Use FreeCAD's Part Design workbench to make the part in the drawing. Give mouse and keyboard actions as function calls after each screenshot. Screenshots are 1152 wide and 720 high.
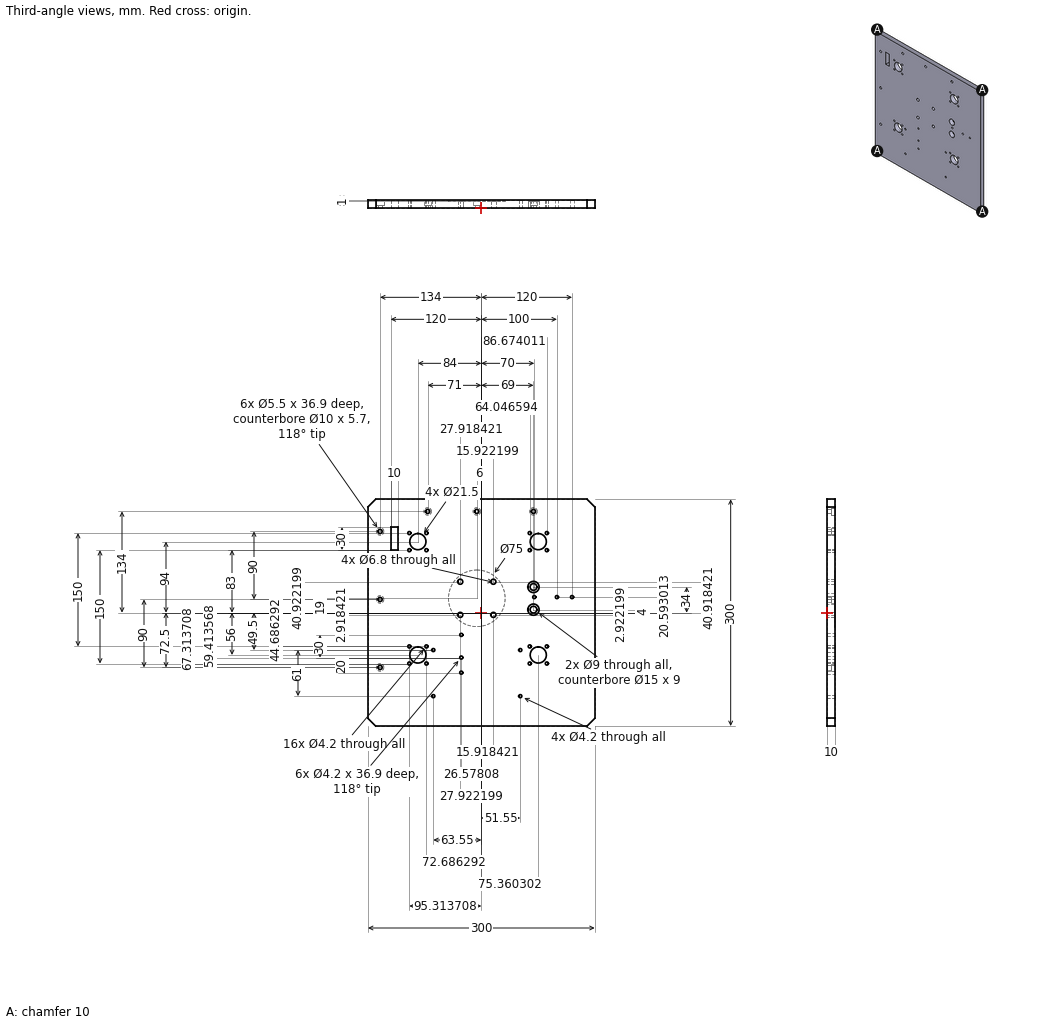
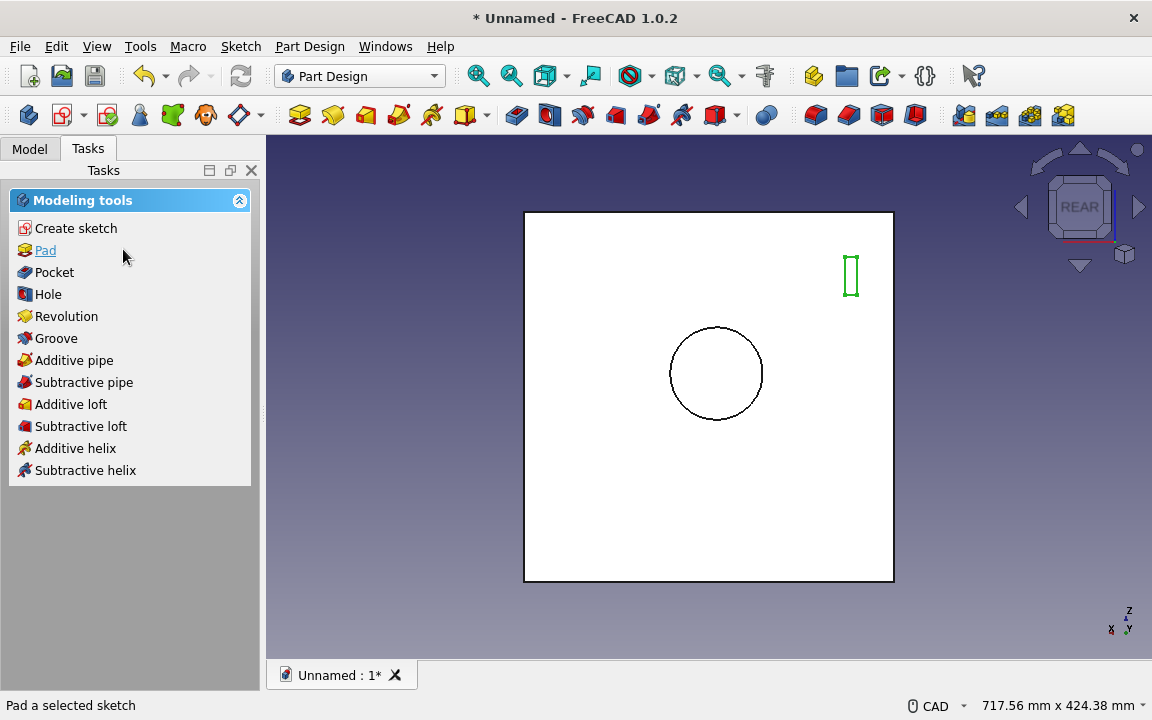
click(517, 116)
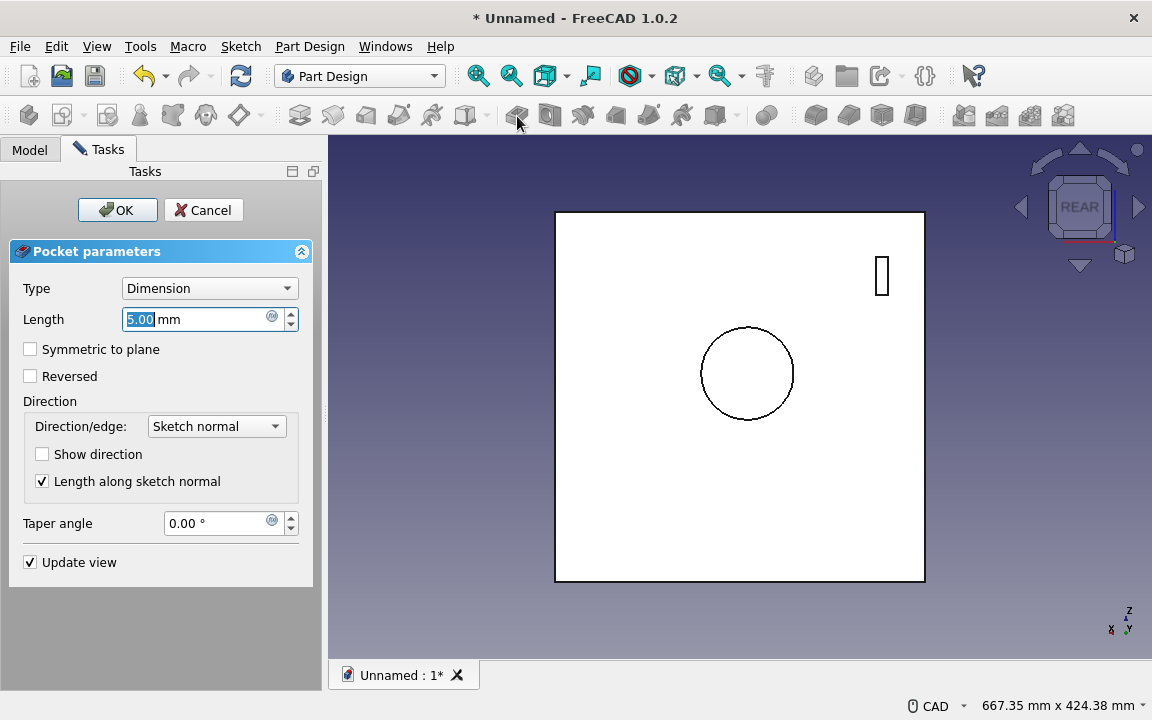
click(210, 288)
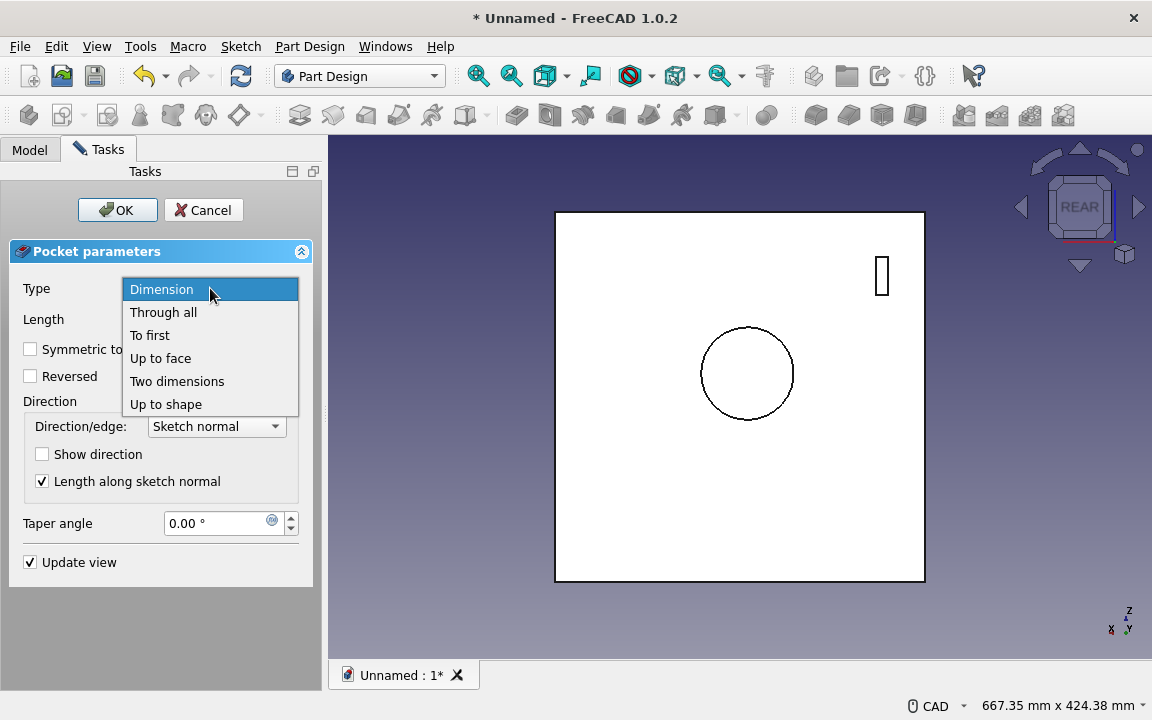
click(208, 312)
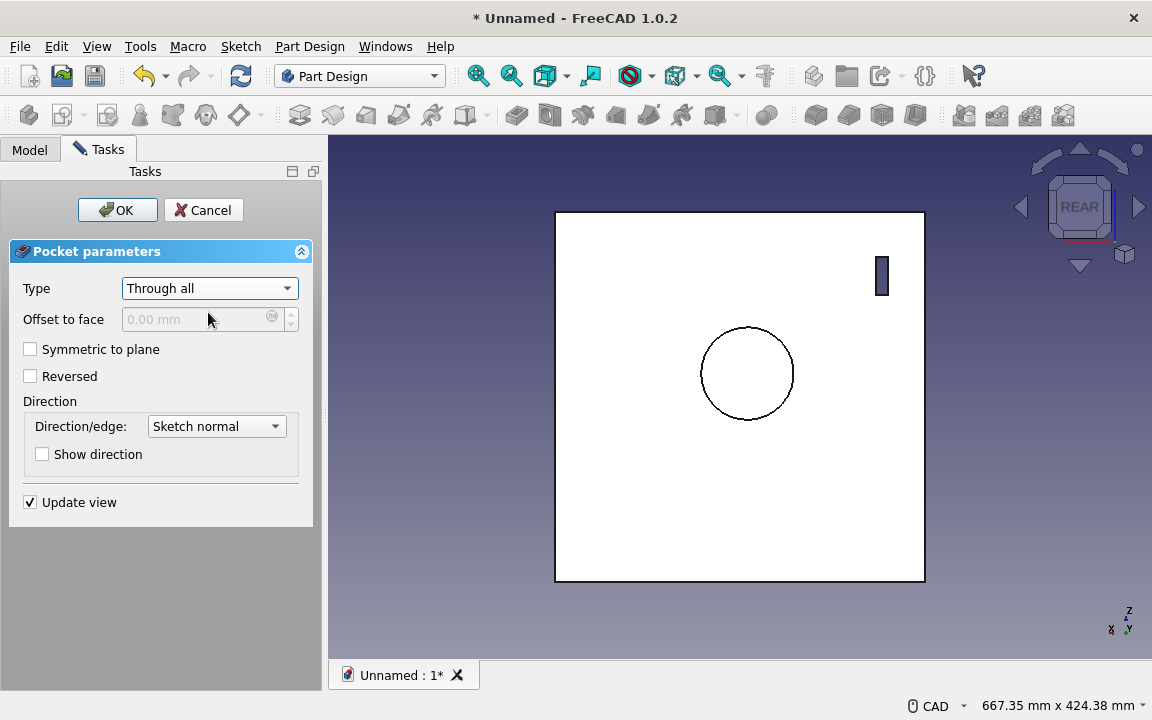
click(118, 210)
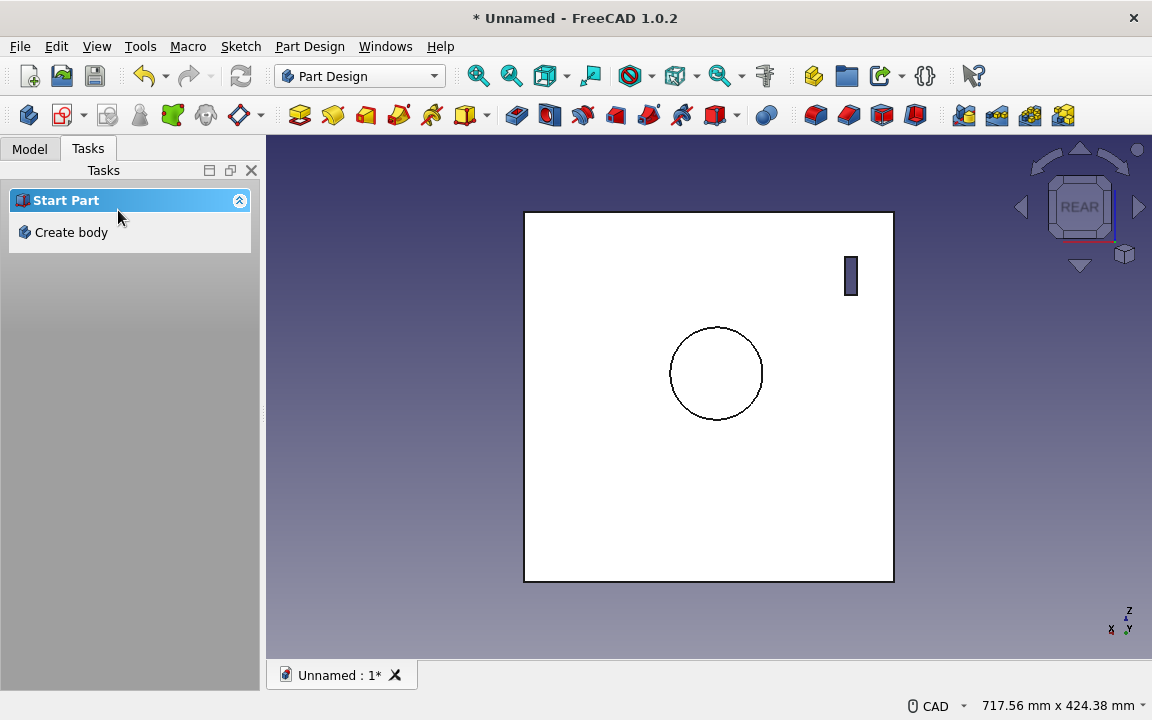
click(656, 502)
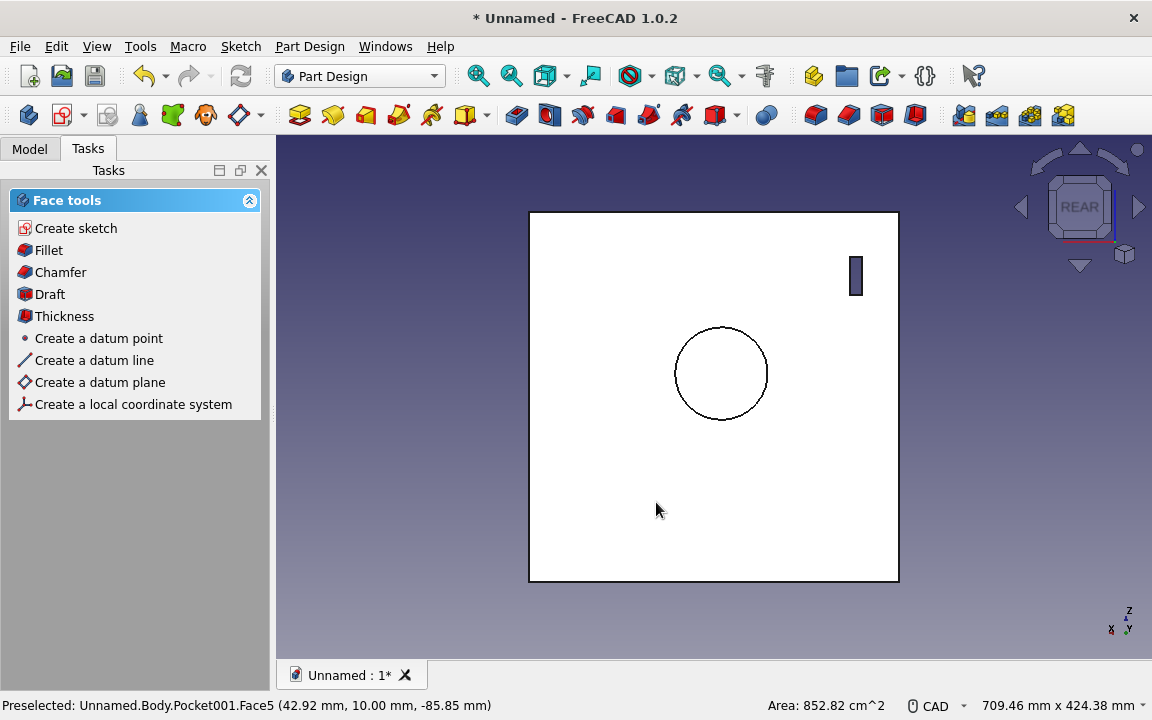
click(62, 116)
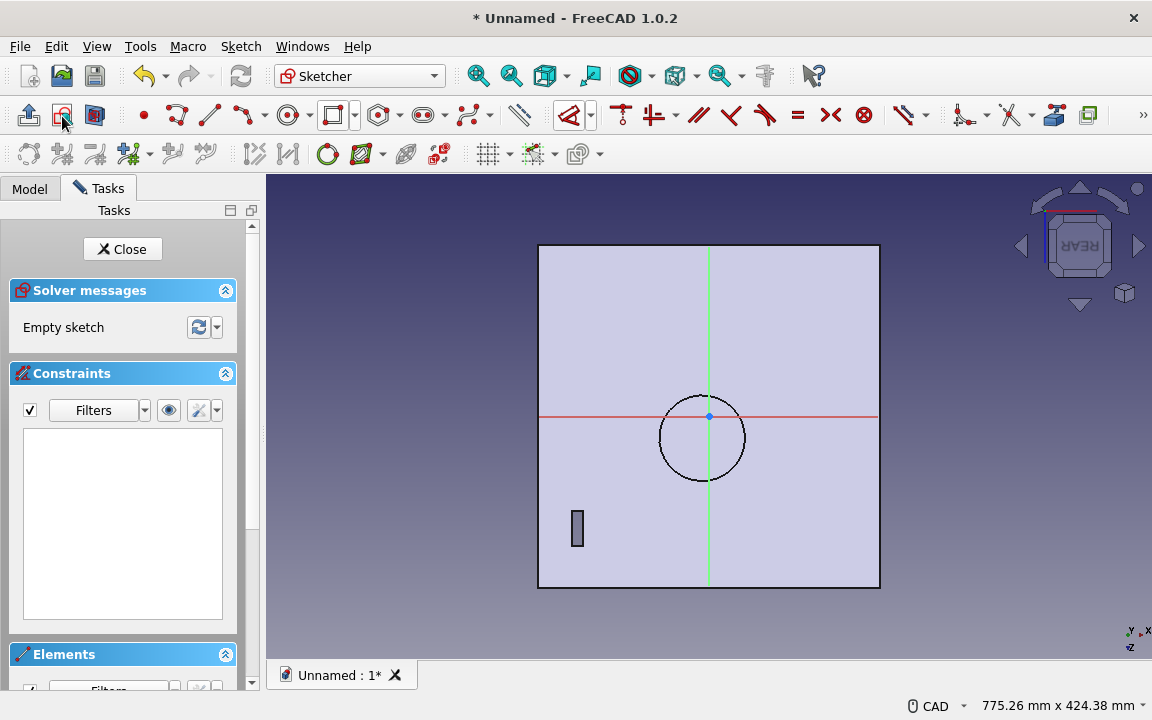
scroll(833, 482, up, 2)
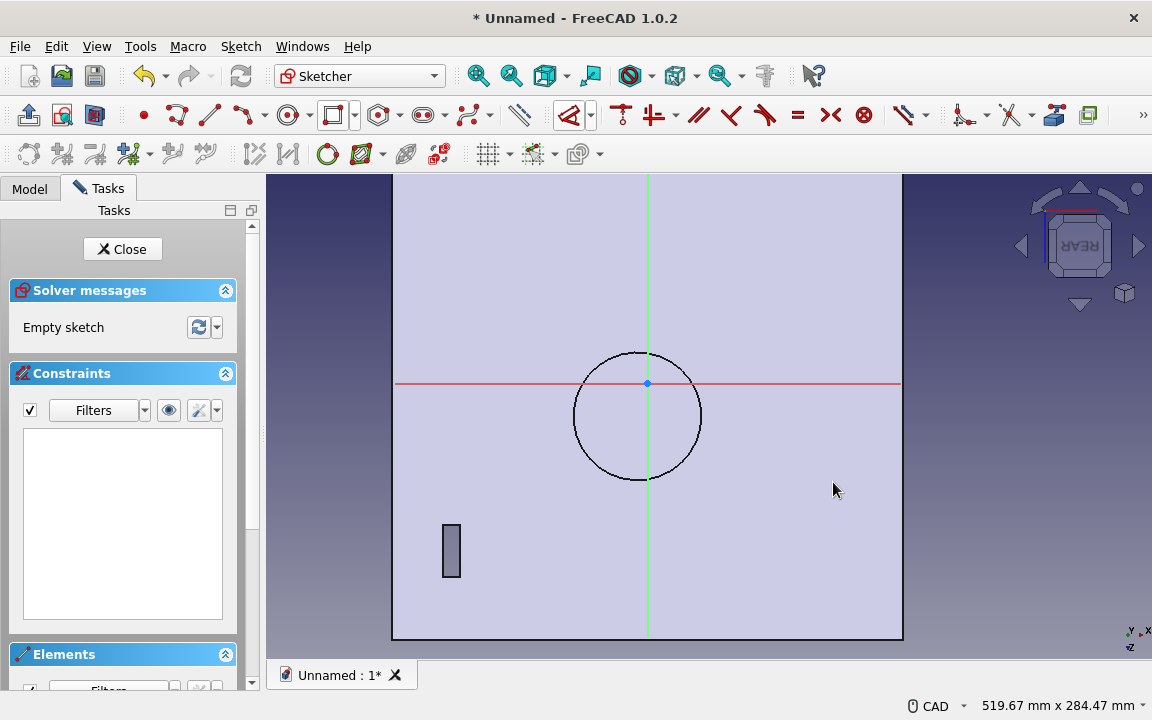
key(g)
key(c)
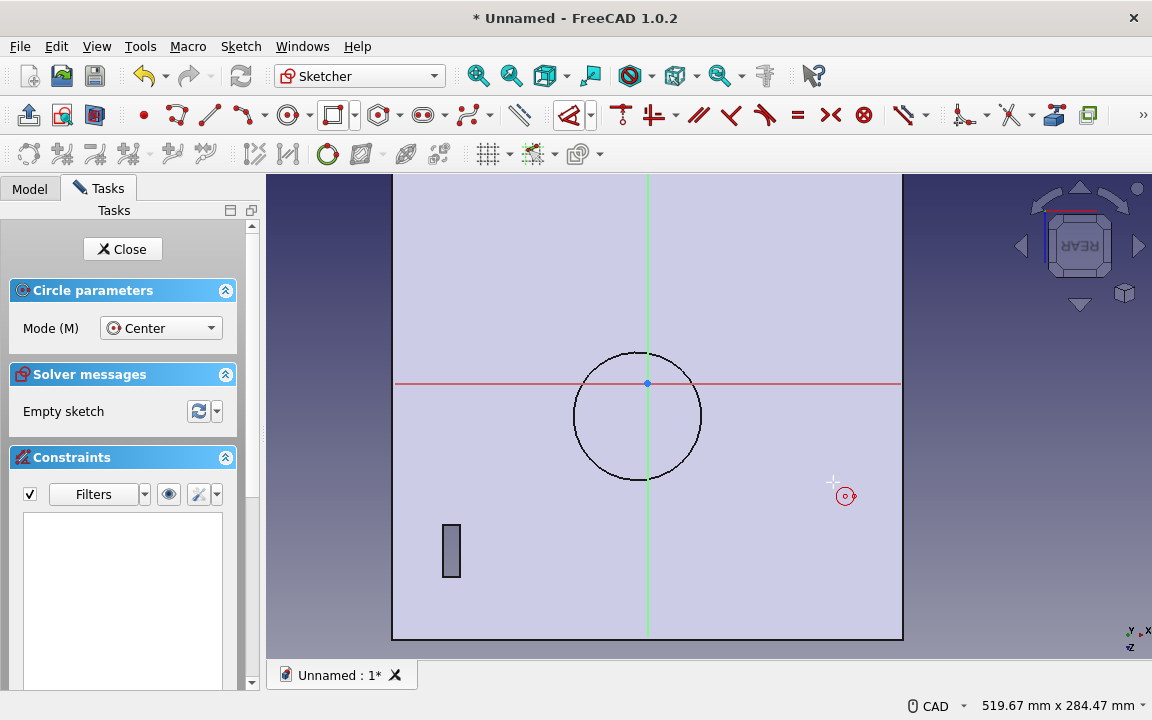
scroll(504, 544, up, 2)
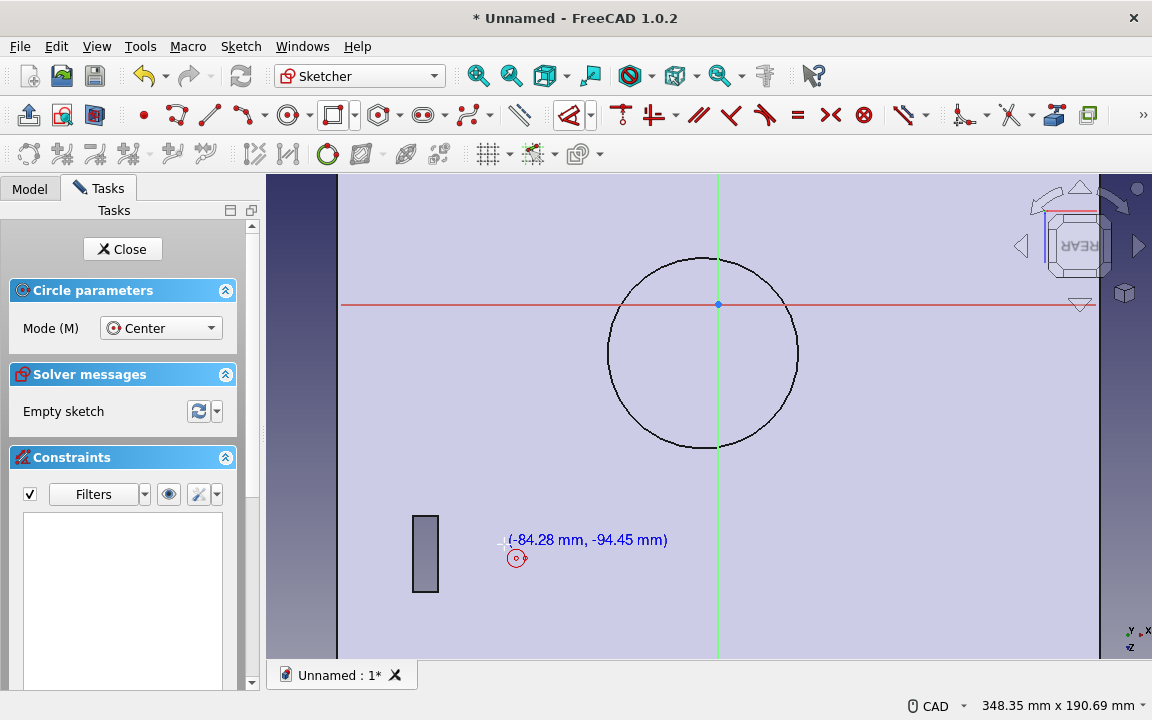
click(505, 544)
move(524, 525)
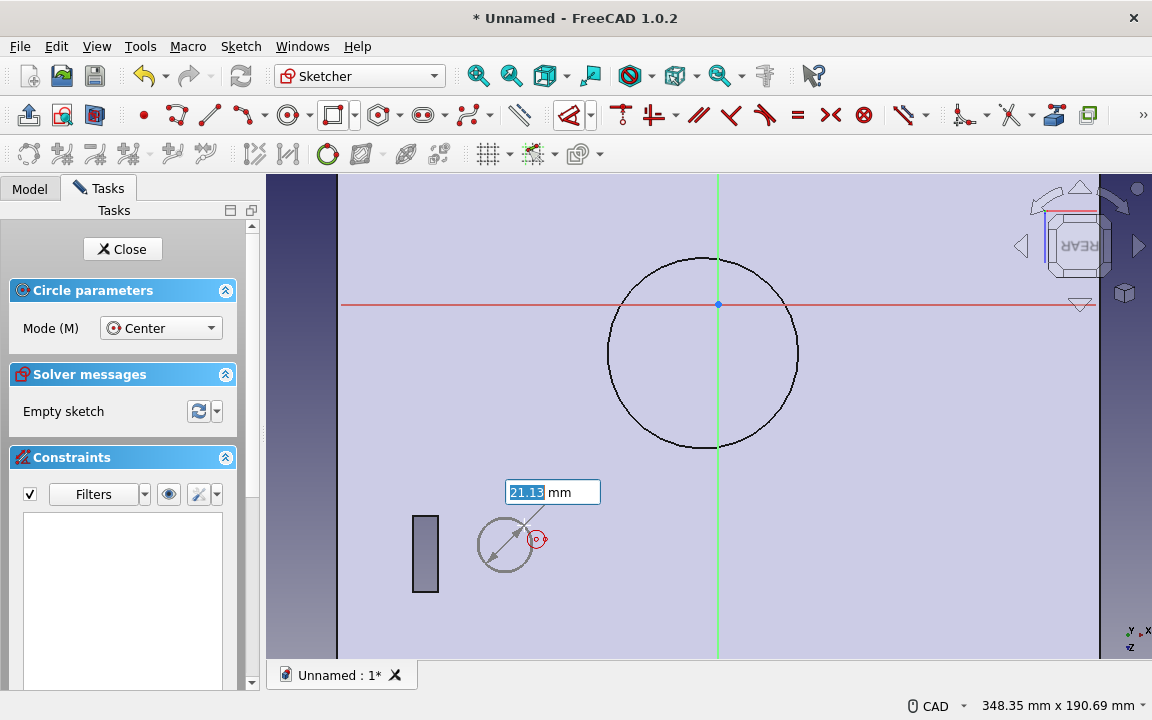
text(21.5)
key(Return)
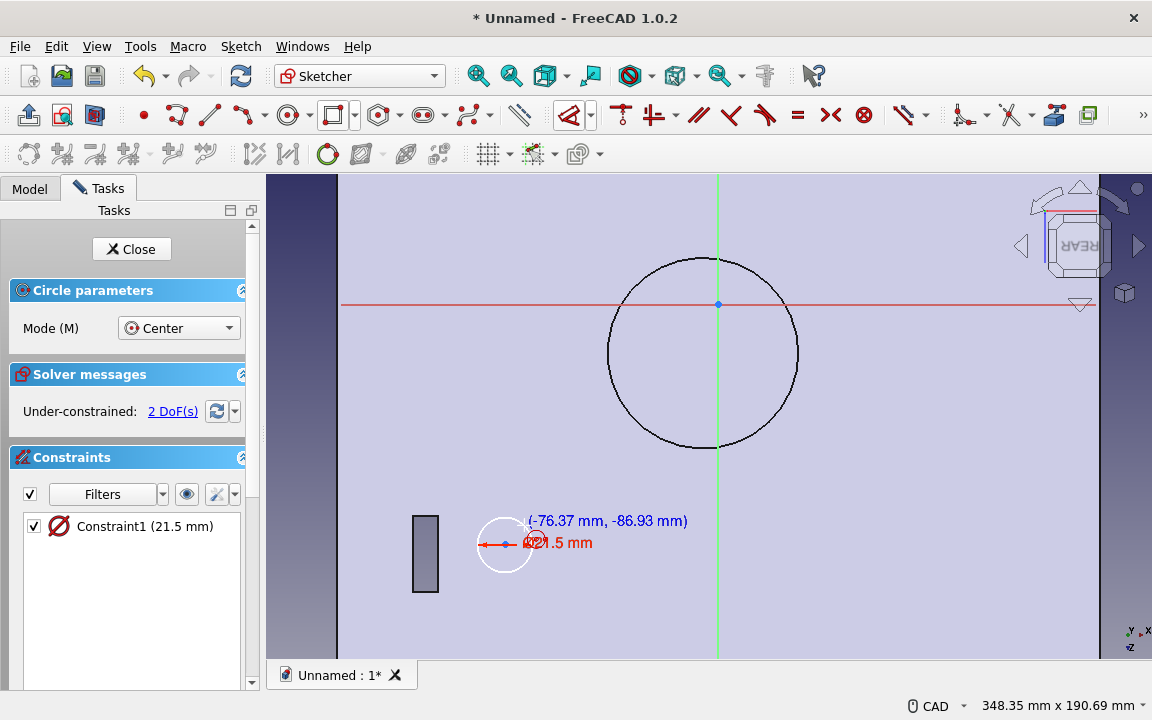
scroll(505, 545, down, 2)